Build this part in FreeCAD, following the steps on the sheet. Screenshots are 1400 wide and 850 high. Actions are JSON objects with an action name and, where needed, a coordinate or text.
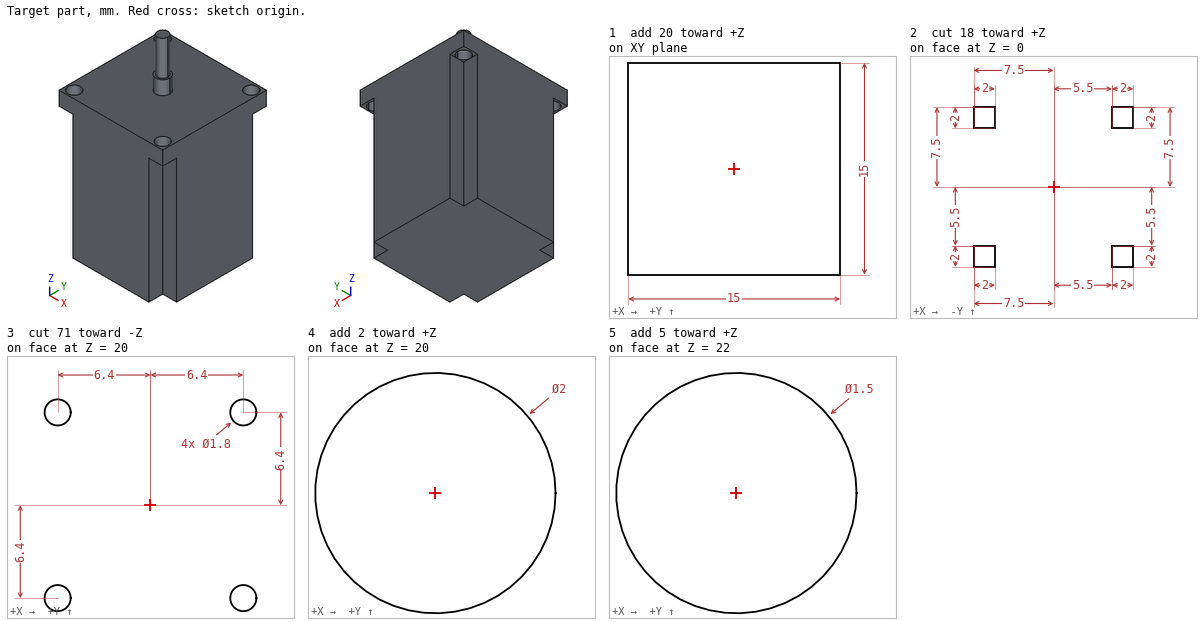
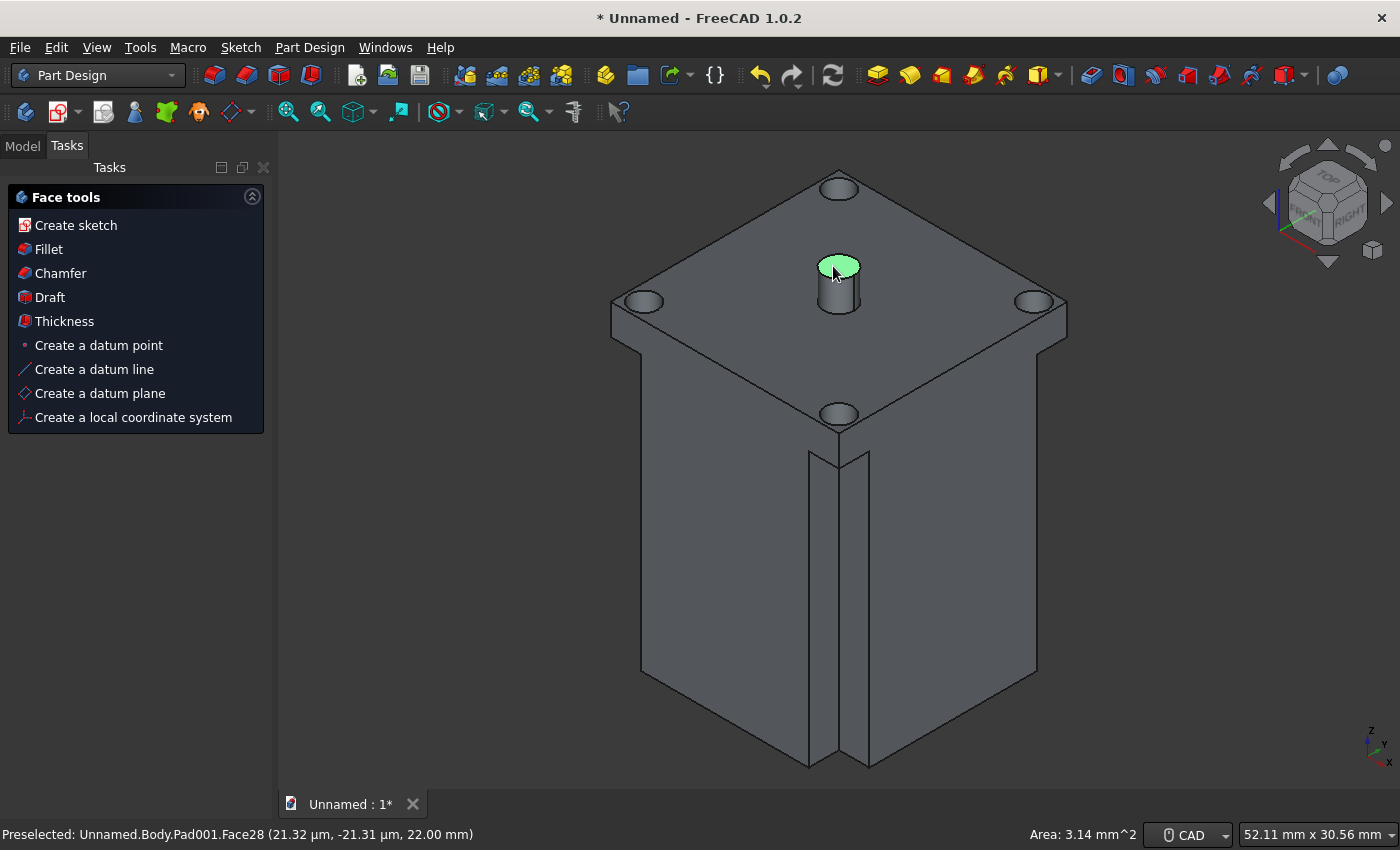
{"action": "left_click", "coordinate": [58, 112]}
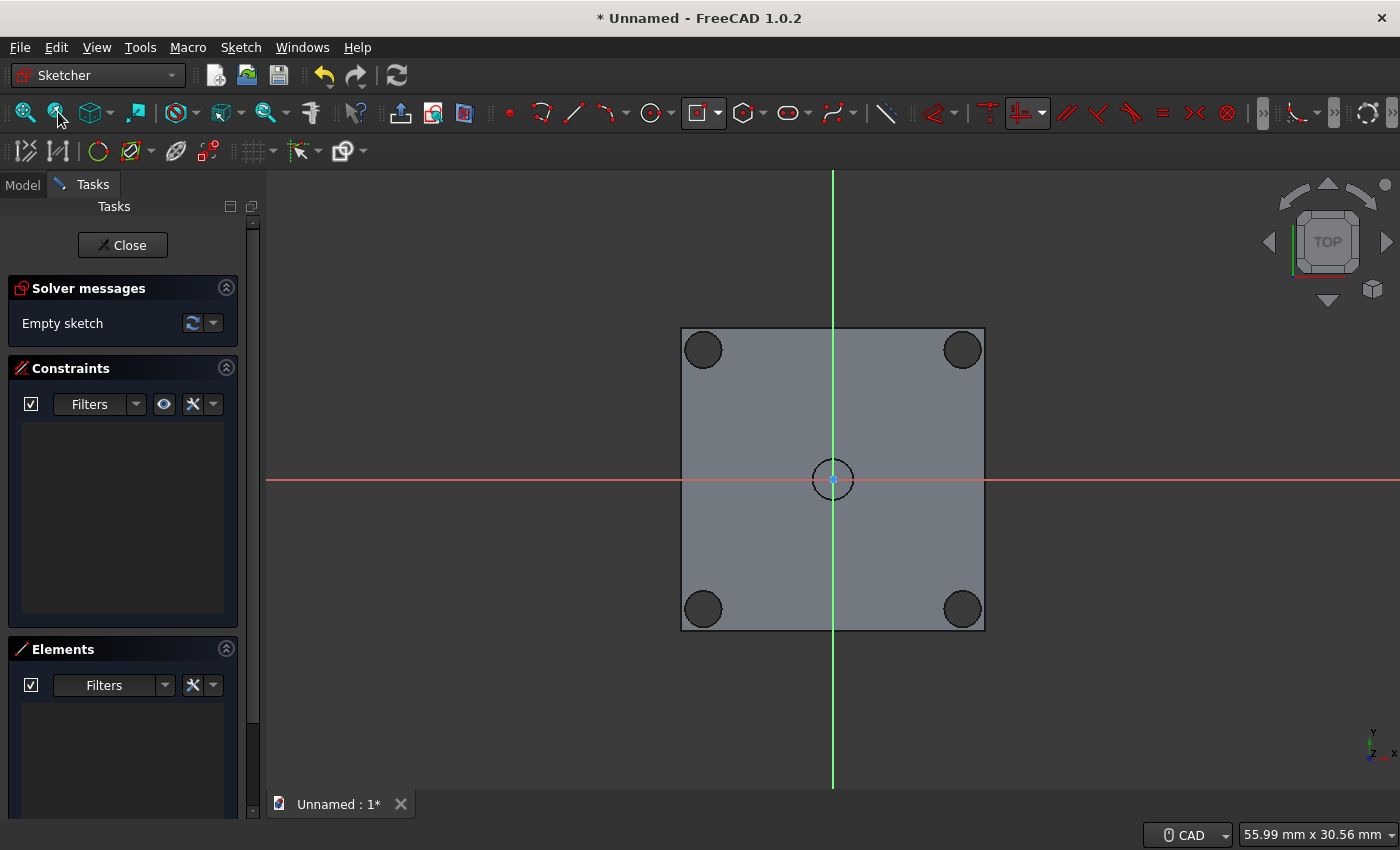
{"action": "scroll", "coordinate": [838, 480], "scroll_direction": "up", "scroll_amount": 13}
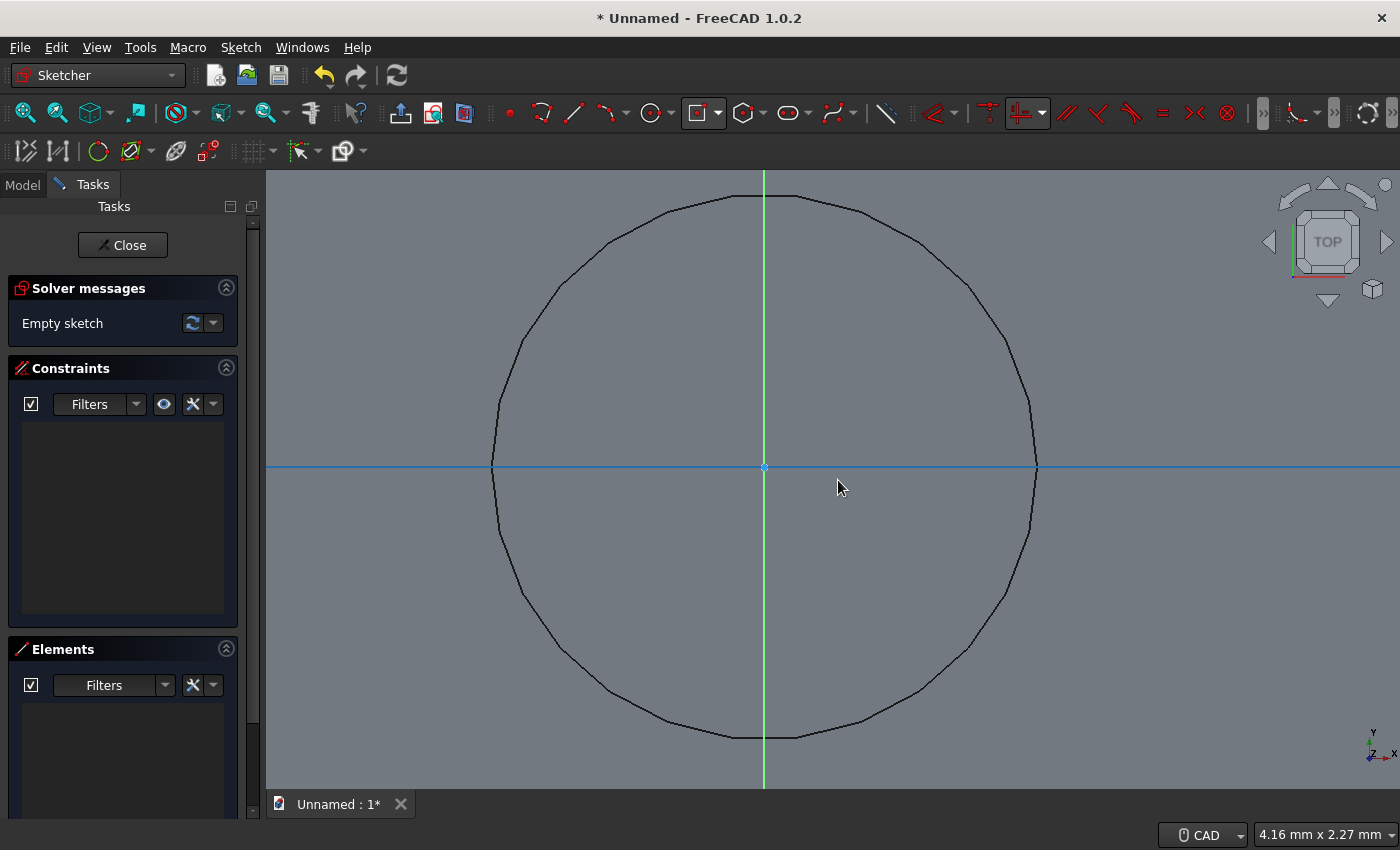
{"action": "left_click", "coordinate": [652, 114]}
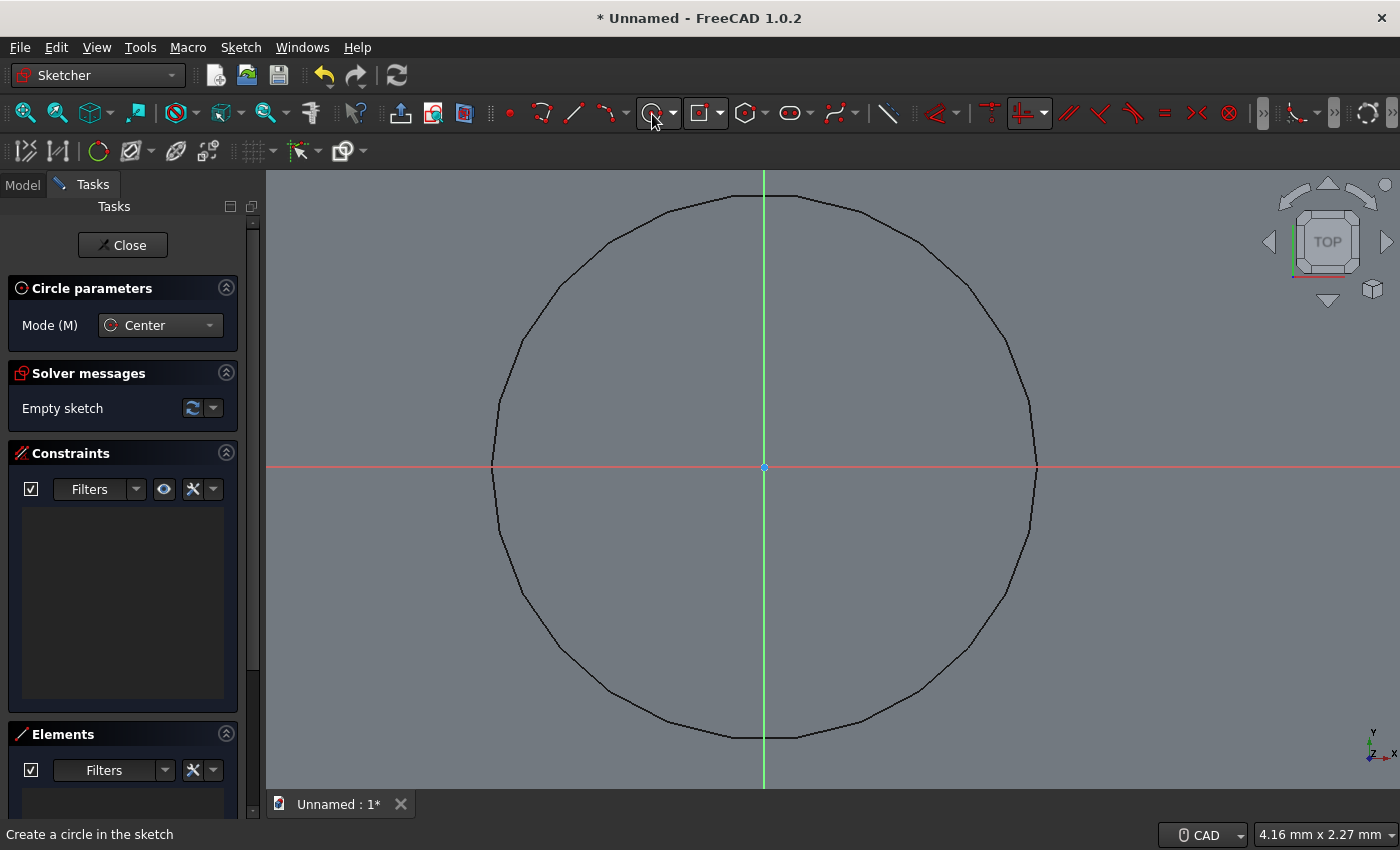
{"action": "left_click", "coordinate": [764, 467]}
{"action": "mouse_move", "coordinate": [909, 322]}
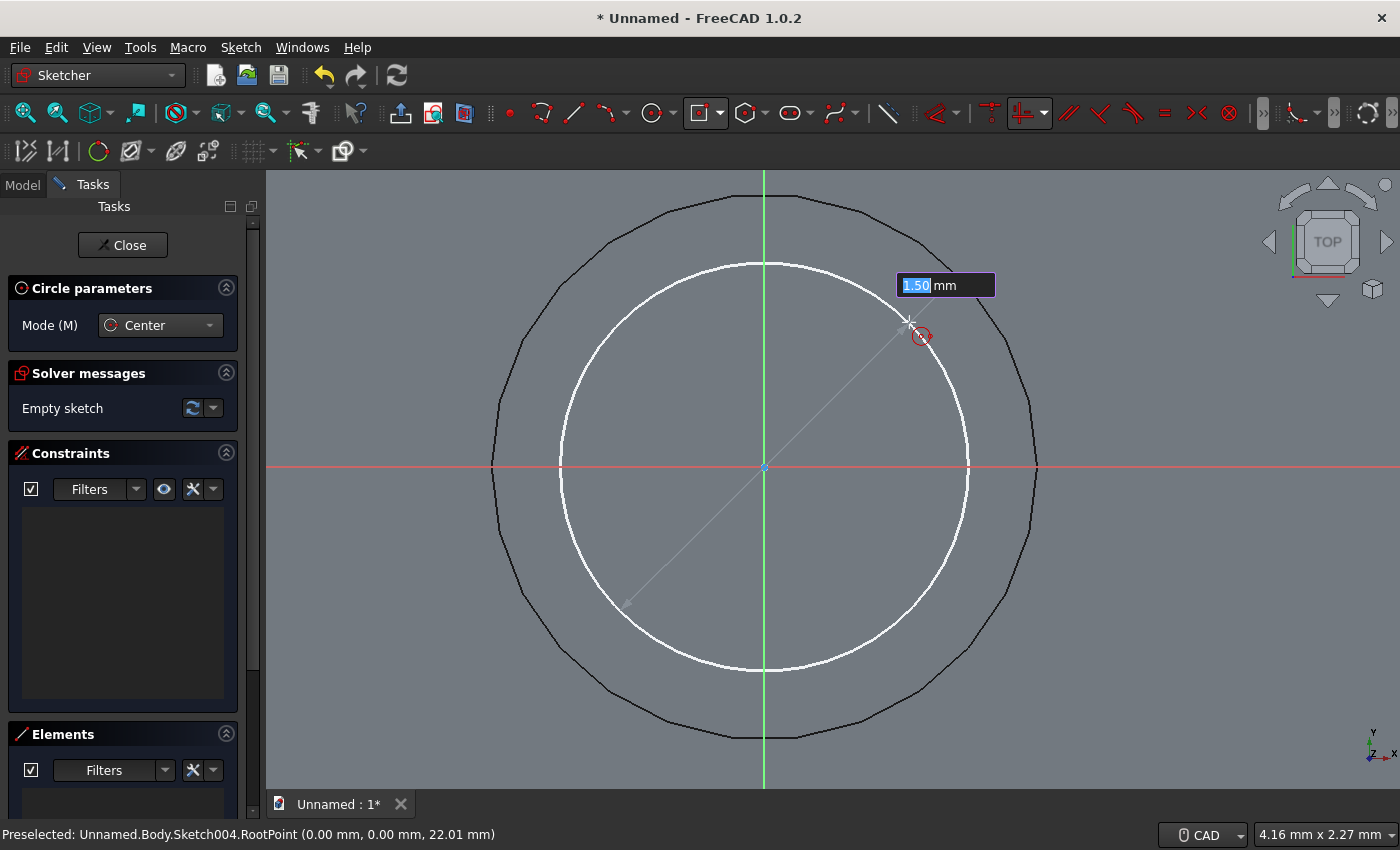
{"action": "type", "text": "1.5"}
{"action": "key", "text": "Return"}
{"action": "key", "text": "Escape"}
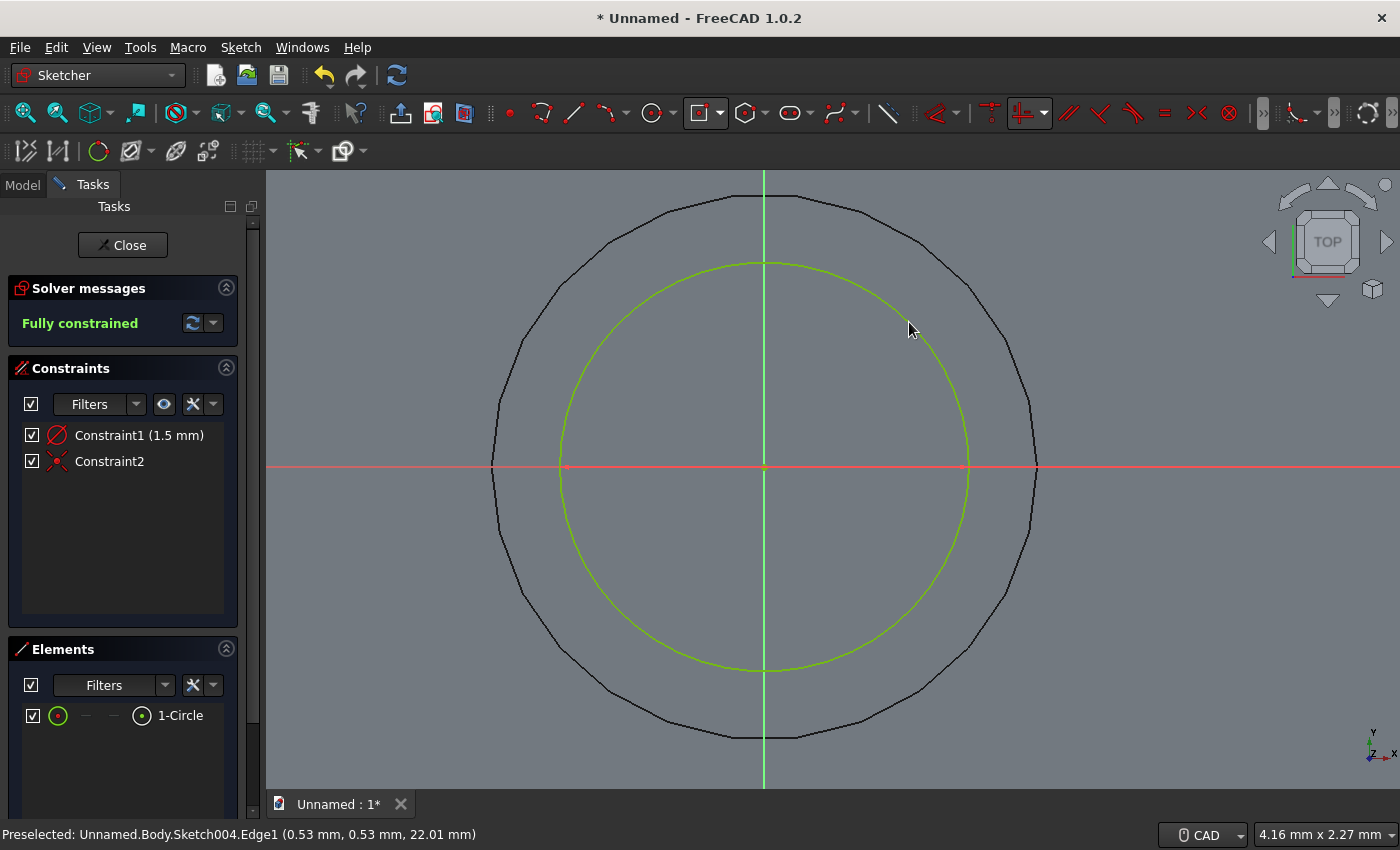
{"action": "left_click", "coordinate": [123, 245]}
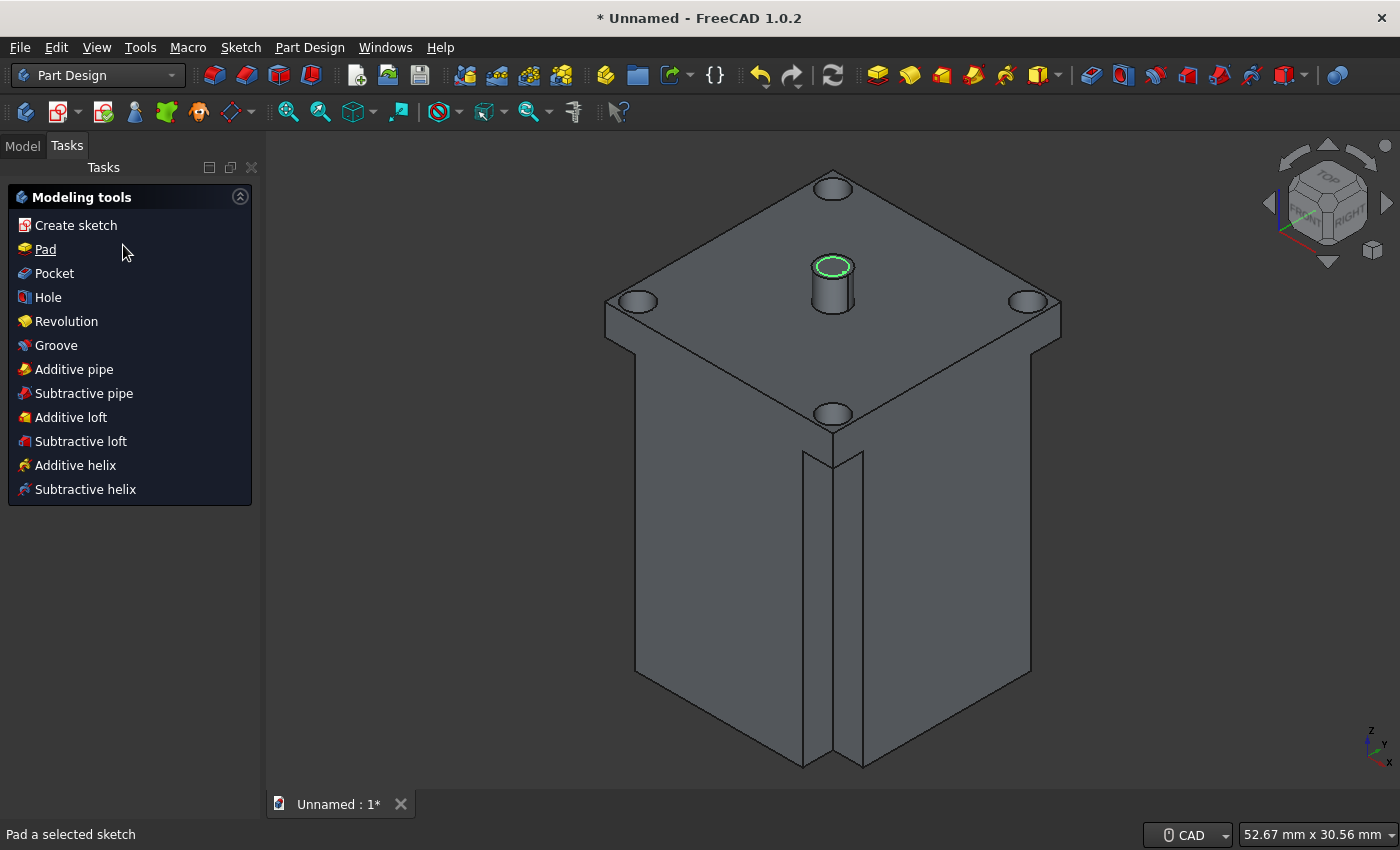
{"action": "left_click", "coordinate": [878, 76]}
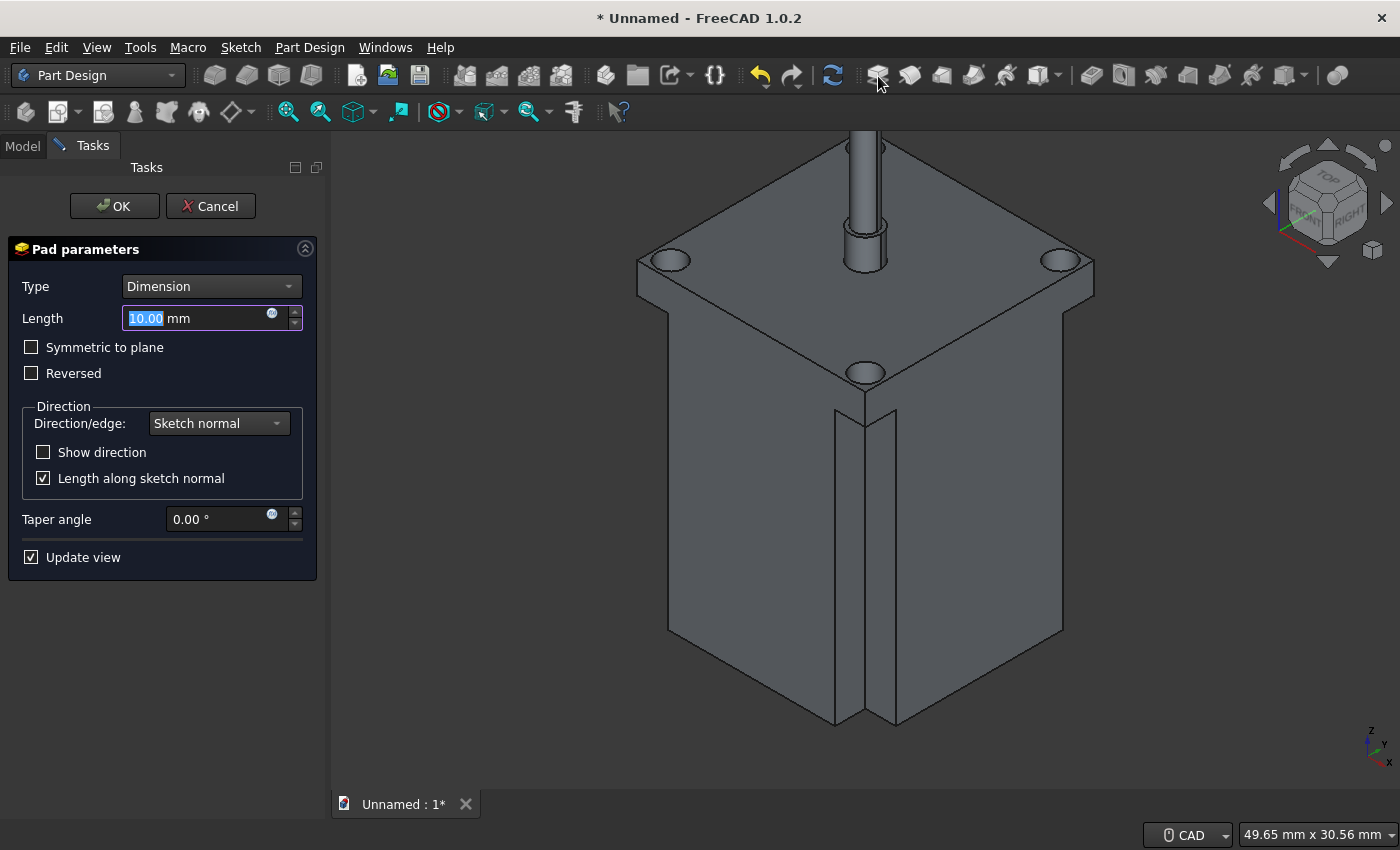
{"action": "type", "text": "5"}
{"action": "key", "text": "Tab"}